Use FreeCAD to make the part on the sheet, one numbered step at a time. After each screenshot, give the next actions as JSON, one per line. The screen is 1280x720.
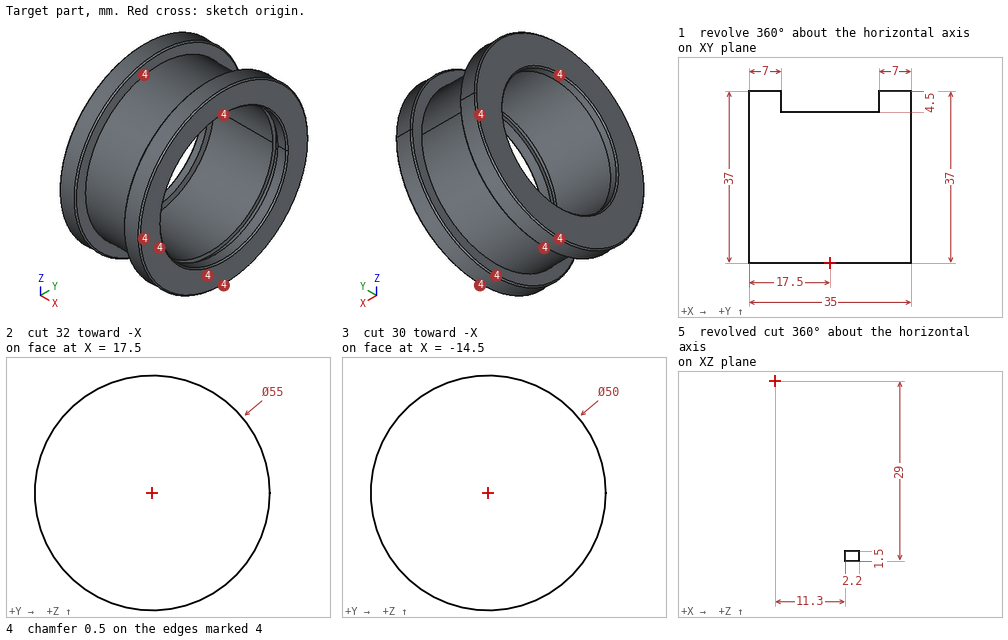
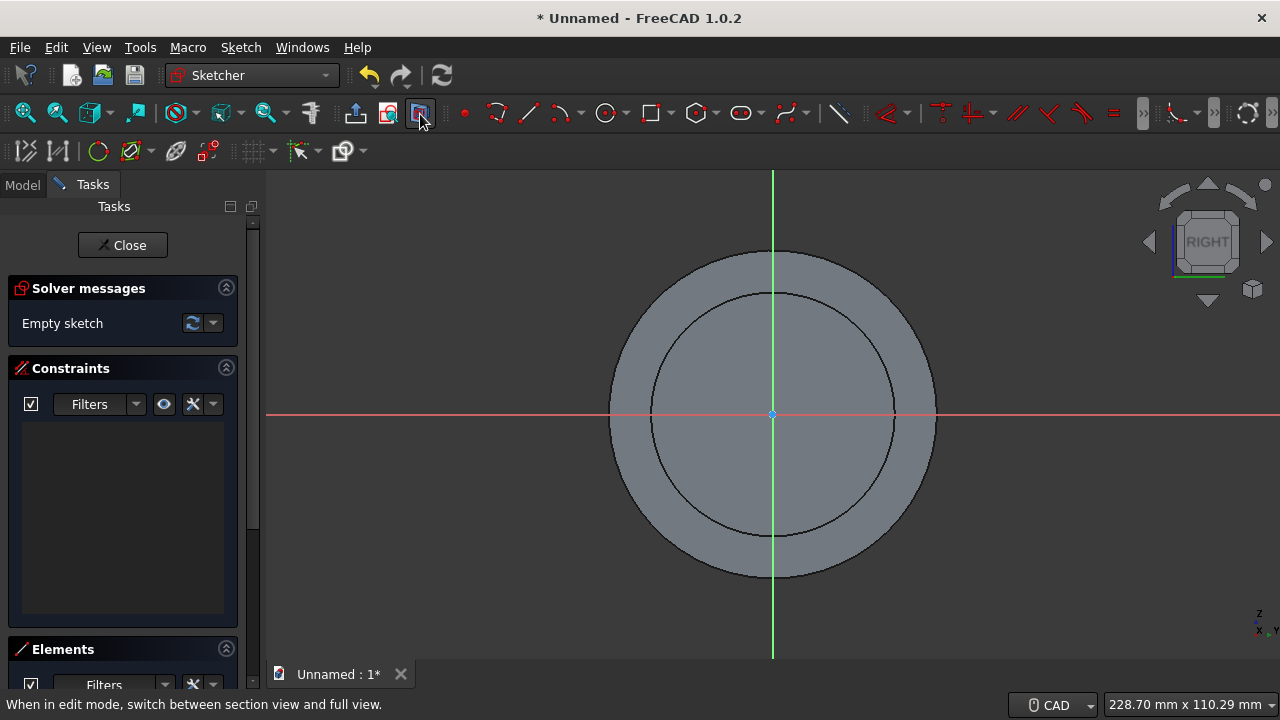
{"action": "scroll", "coordinate": [912, 414], "scroll_direction": "up", "scroll_amount": 2}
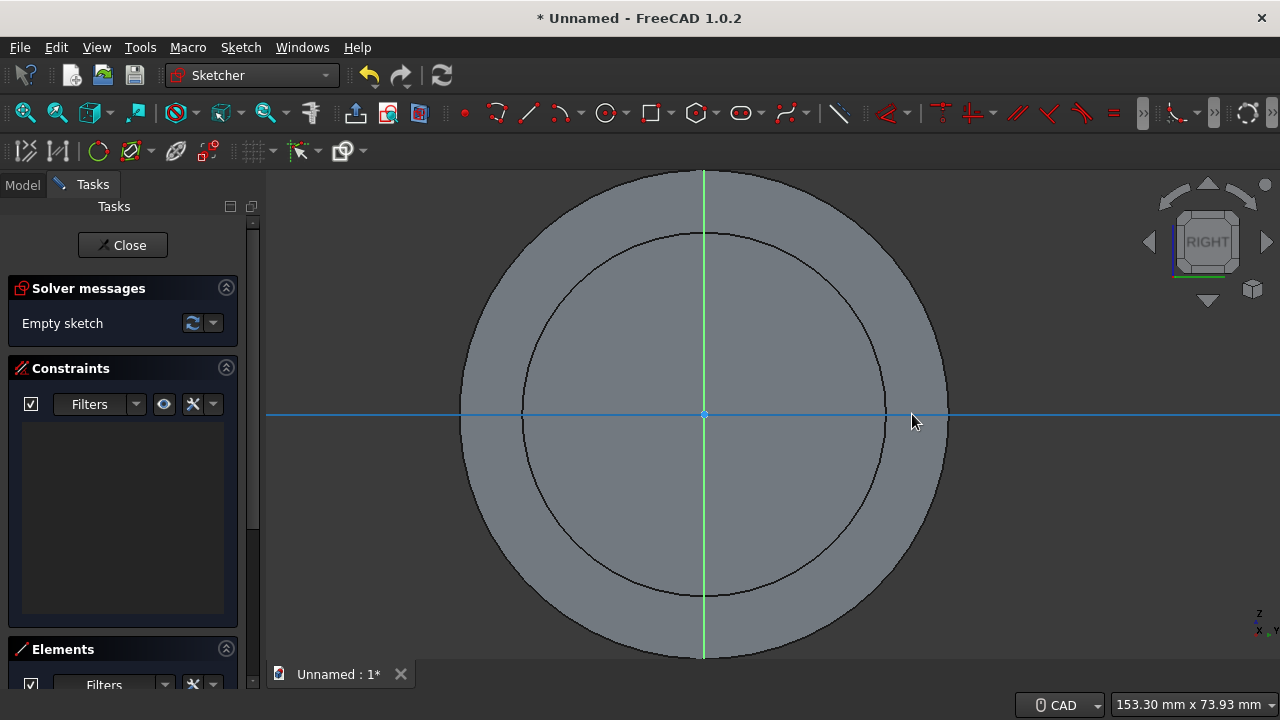
{"action": "key", "text": "g c"}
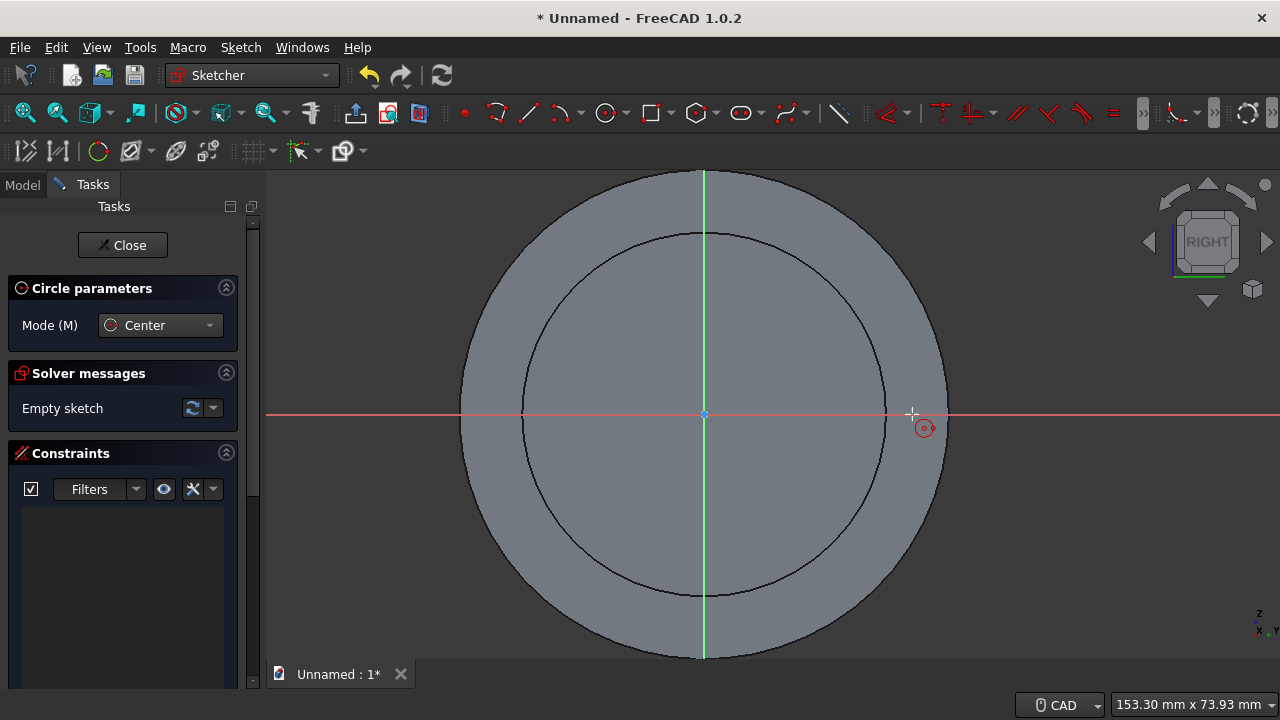
{"action": "left_click", "coordinate": [704, 414]}
{"action": "left_click", "coordinate": [821, 298]}
{"action": "key", "text": "Escape"}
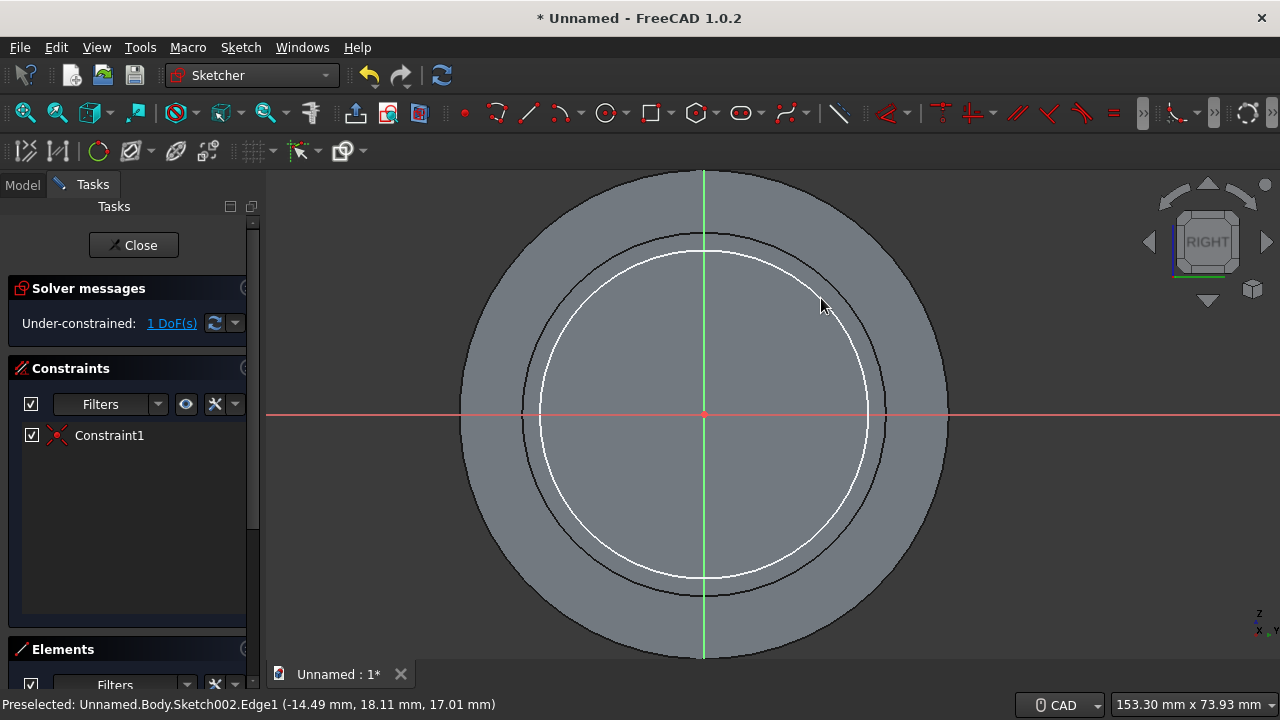
{"action": "left_click", "coordinate": [886, 114]}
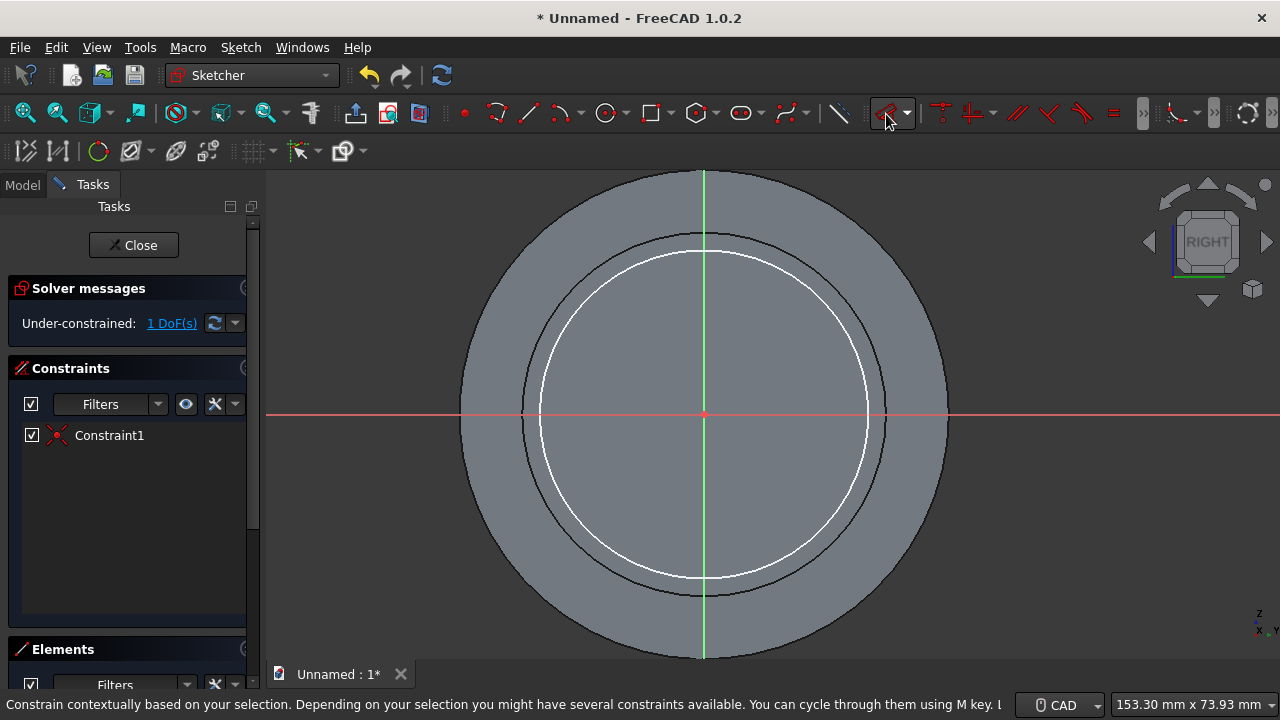
{"action": "left_click", "coordinate": [820, 298]}
{"action": "left_click", "coordinate": [843, 275]}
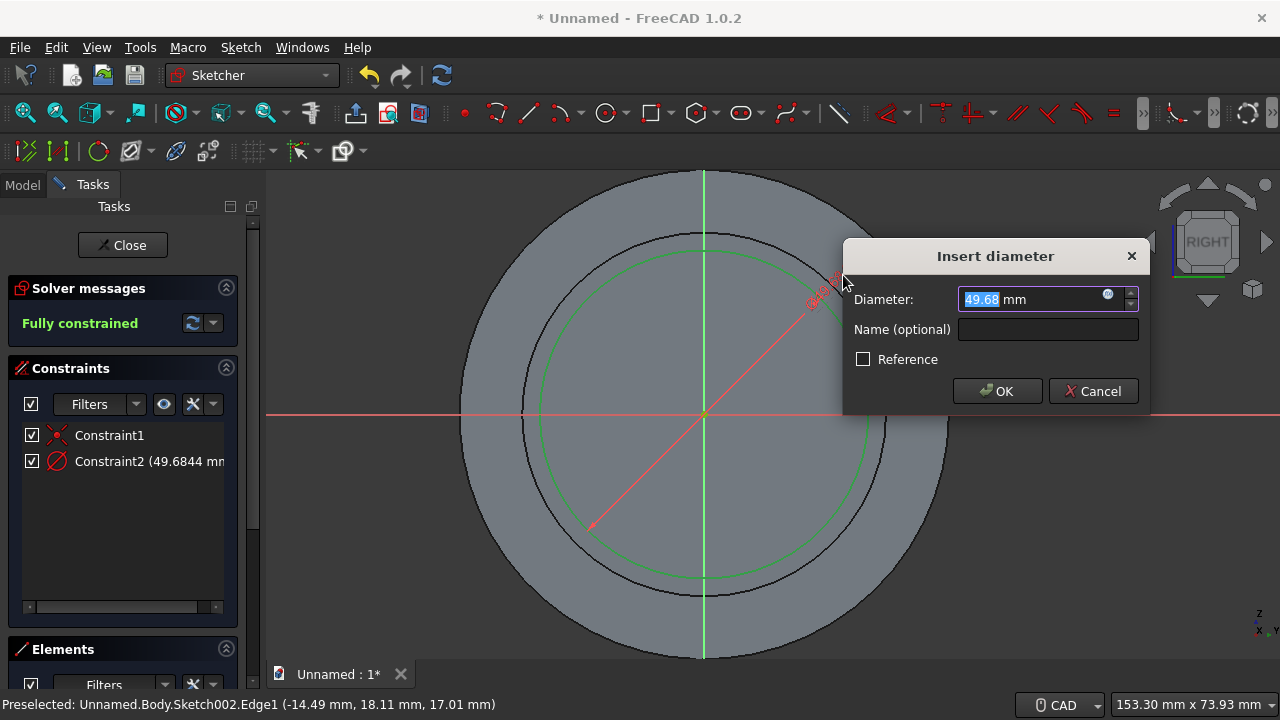
{"action": "type", "text": "50"}
{"action": "key", "text": "Return"}
{"action": "key", "text": "Escape"}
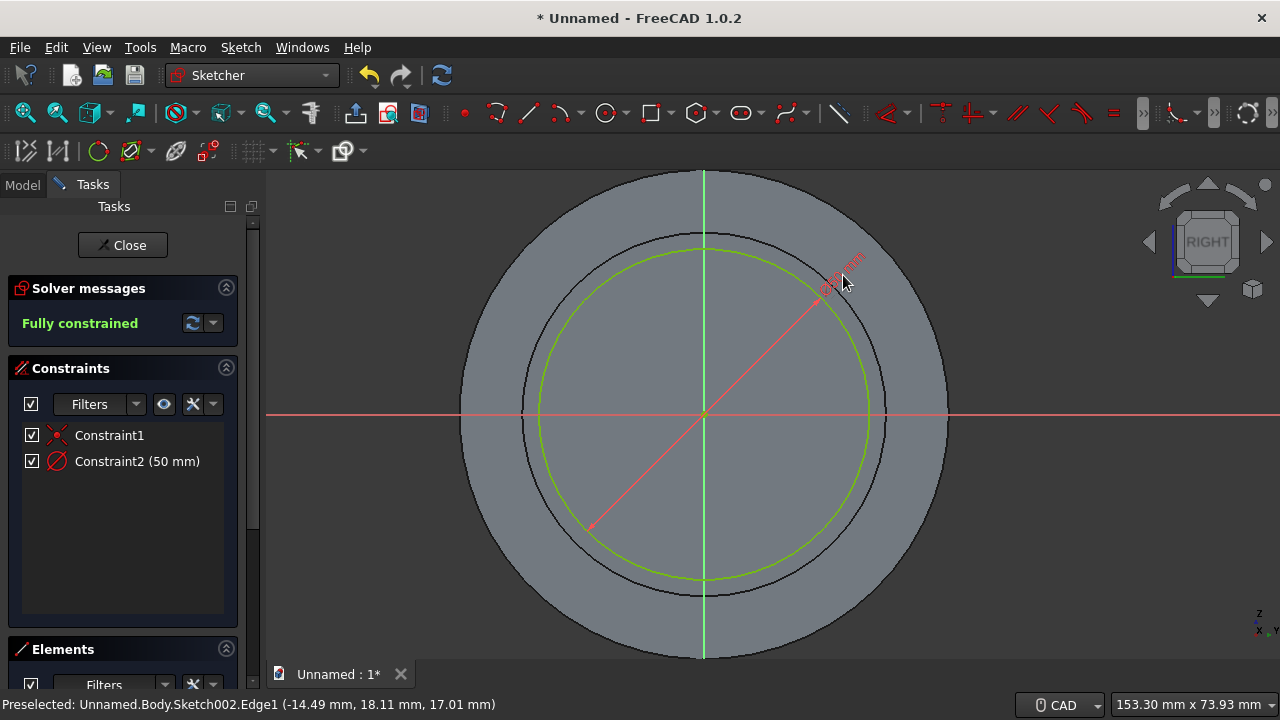
{"action": "left_click", "coordinate": [123, 245]}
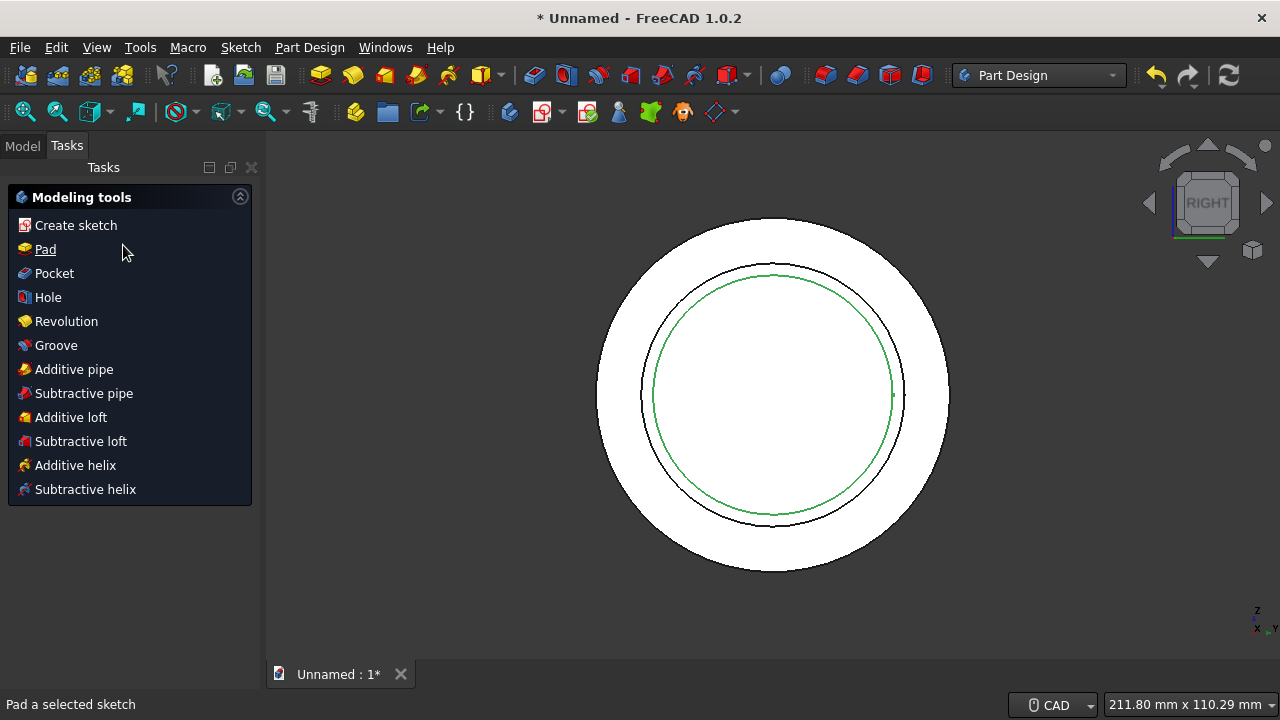
{"action": "left_click", "coordinate": [536, 76]}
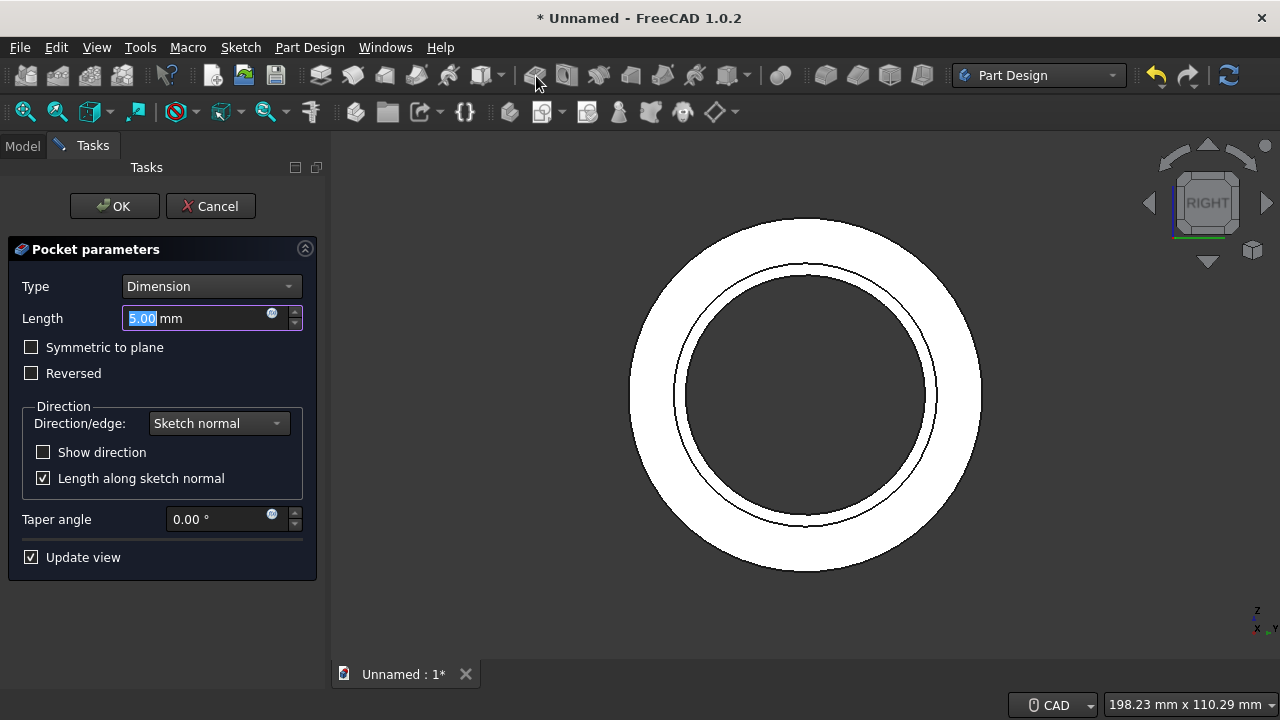
{"action": "type", "text": "30"}
{"action": "key", "text": "Tab"}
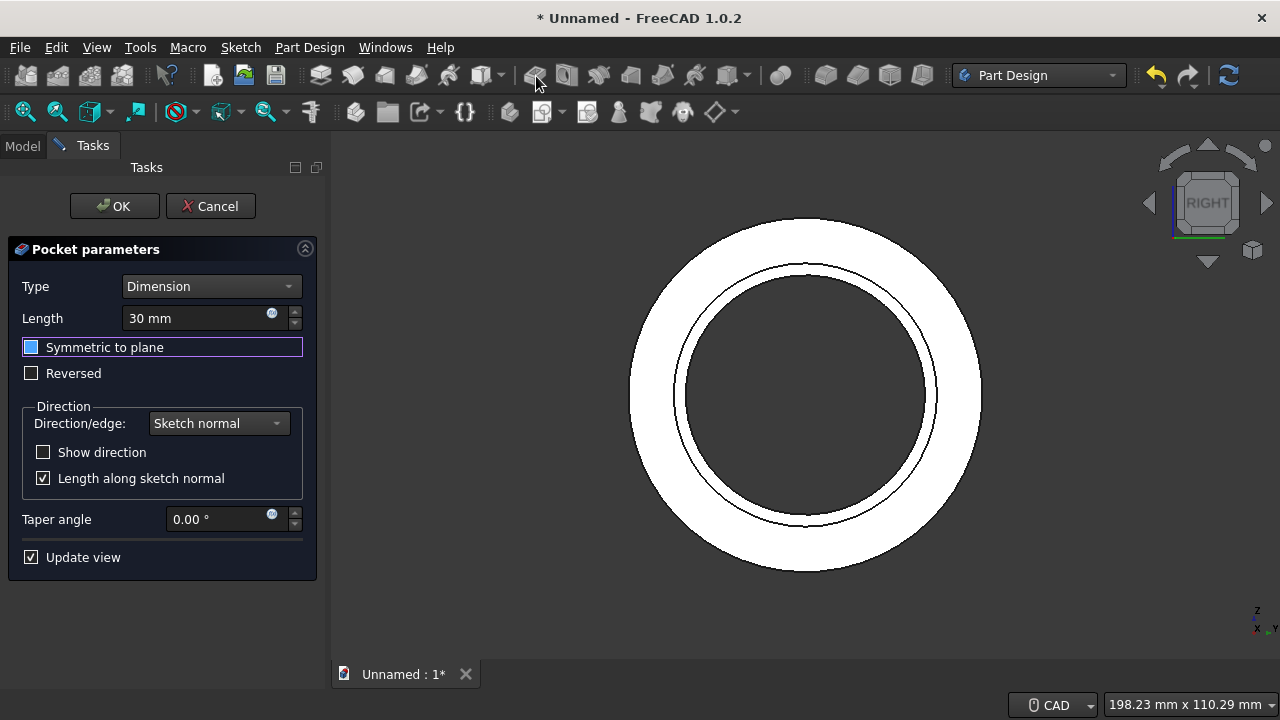
{"action": "left_click", "coordinate": [115, 206]}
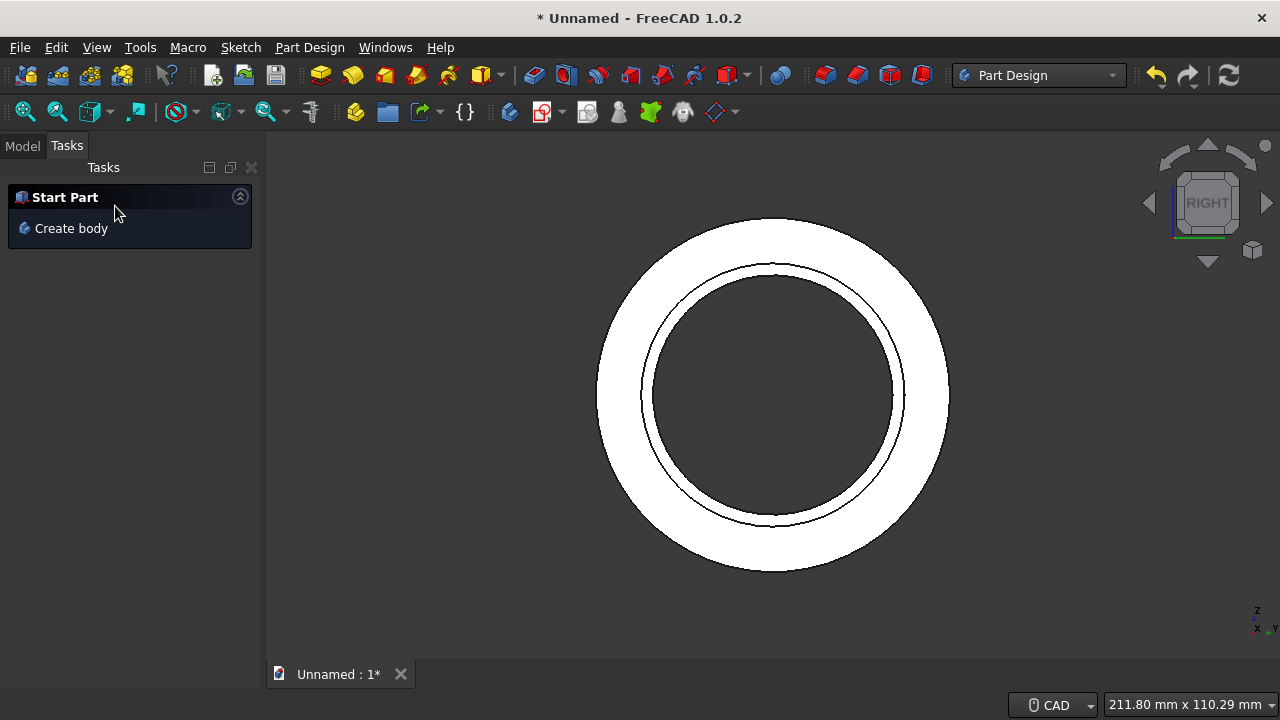
{"action": "left_click", "coordinate": [641, 394]}